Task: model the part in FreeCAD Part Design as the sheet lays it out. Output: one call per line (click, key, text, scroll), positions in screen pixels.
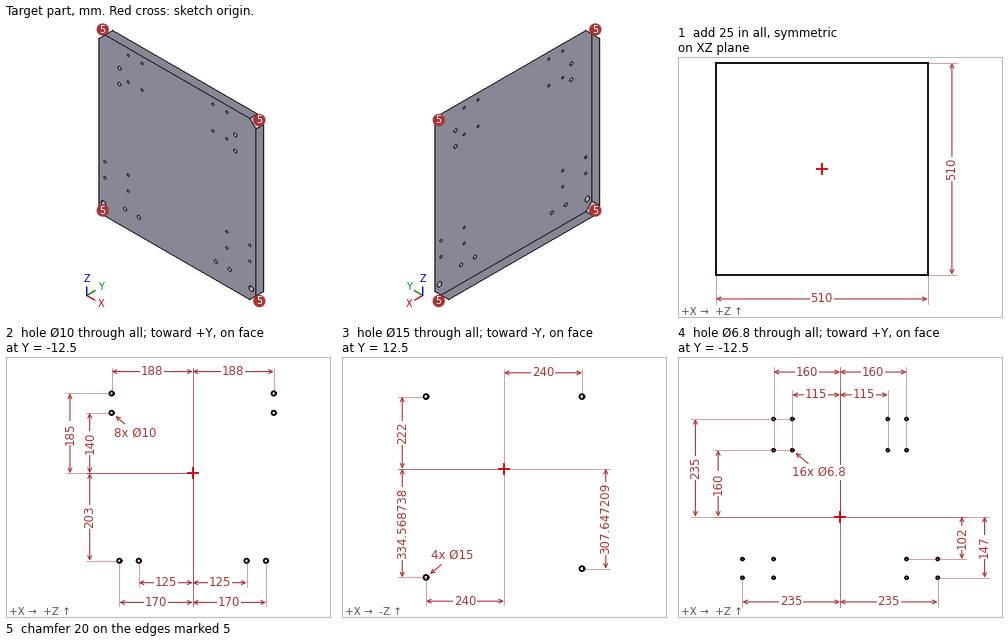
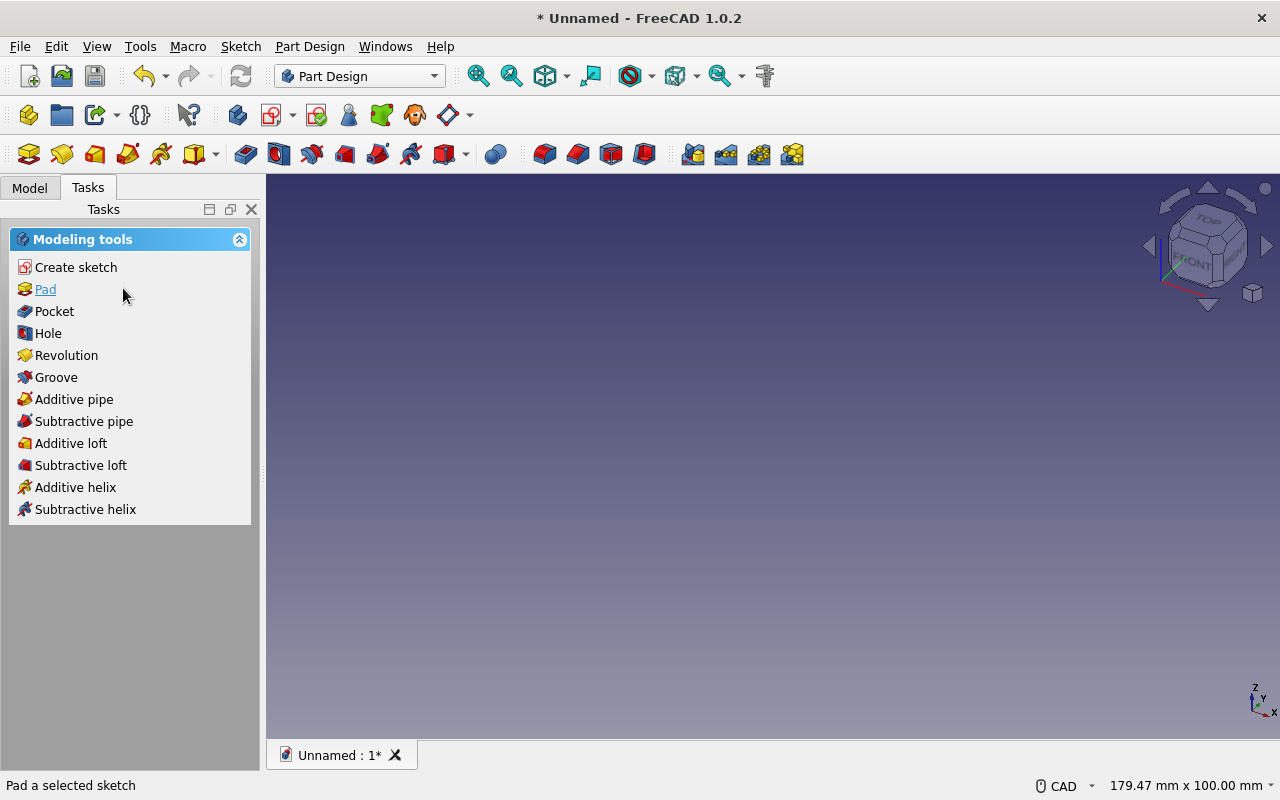
click(29, 154)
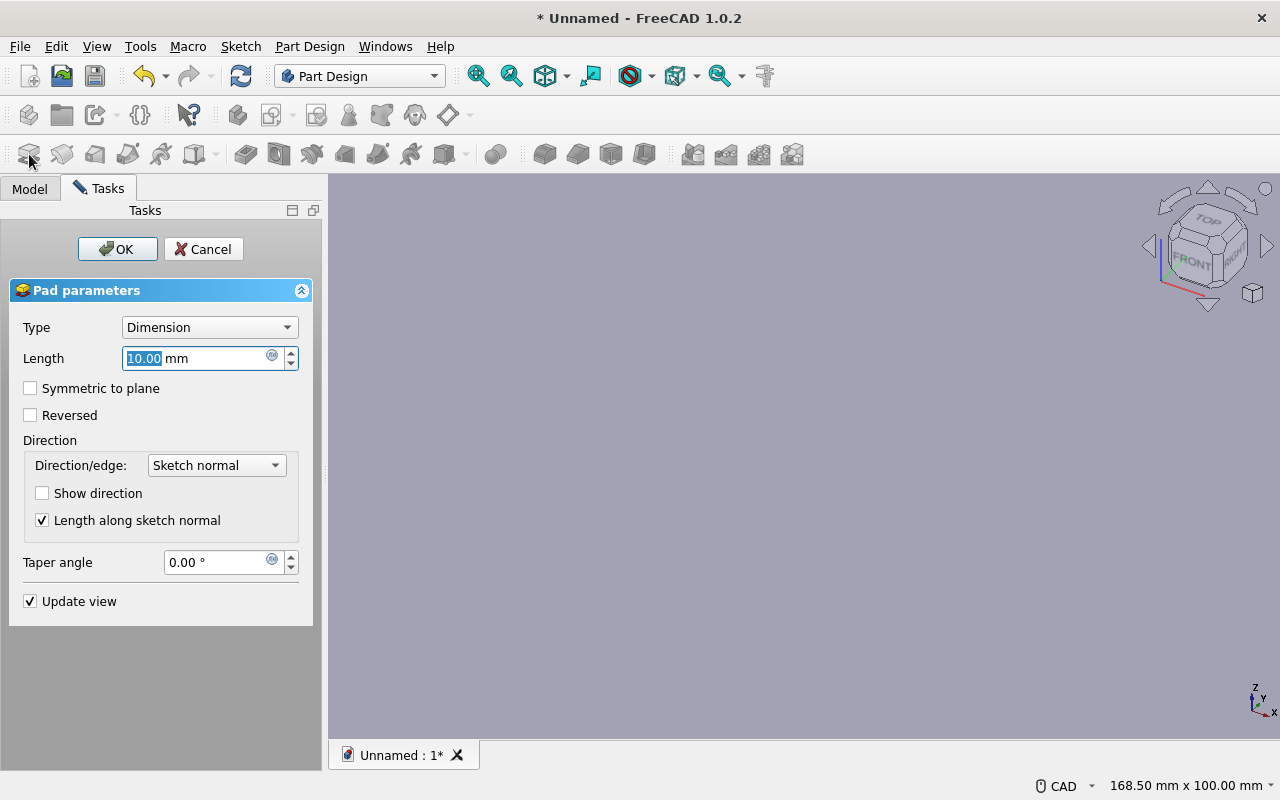
text(25)
key(Tab)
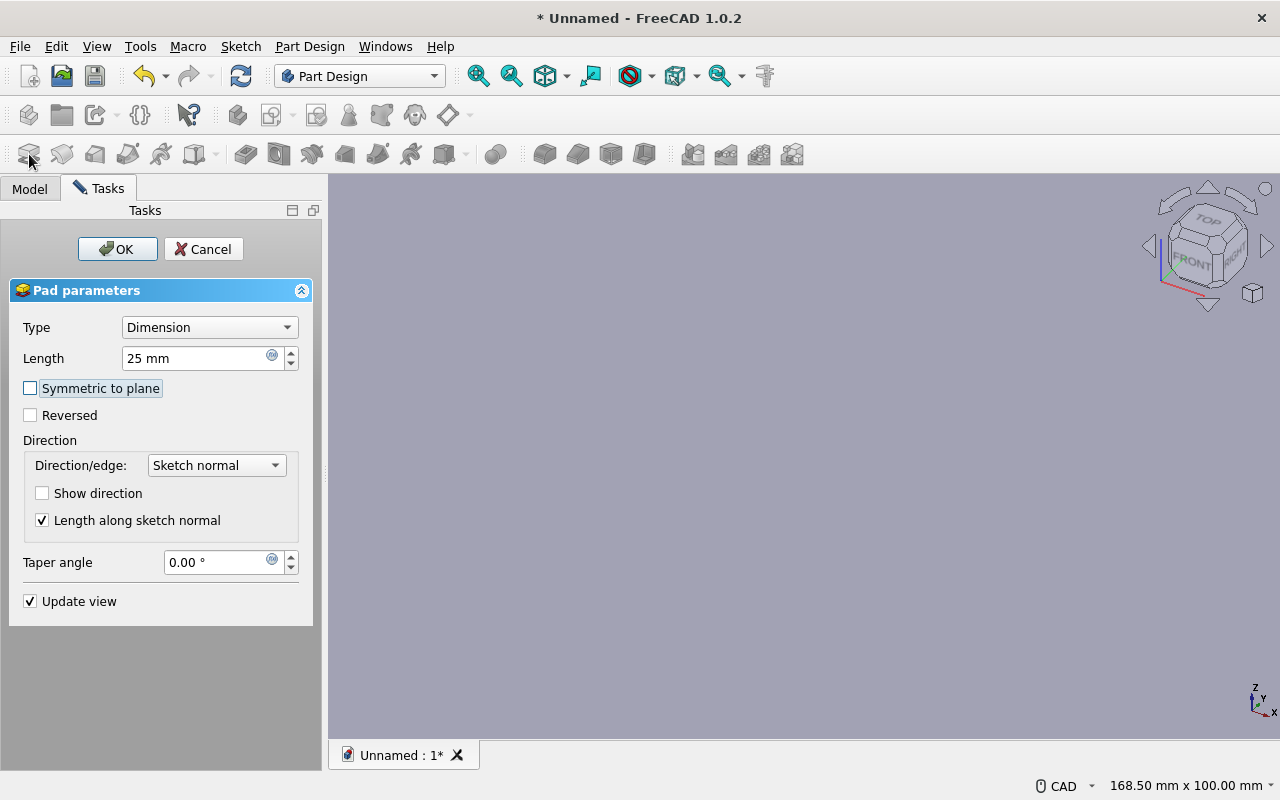
click(31, 388)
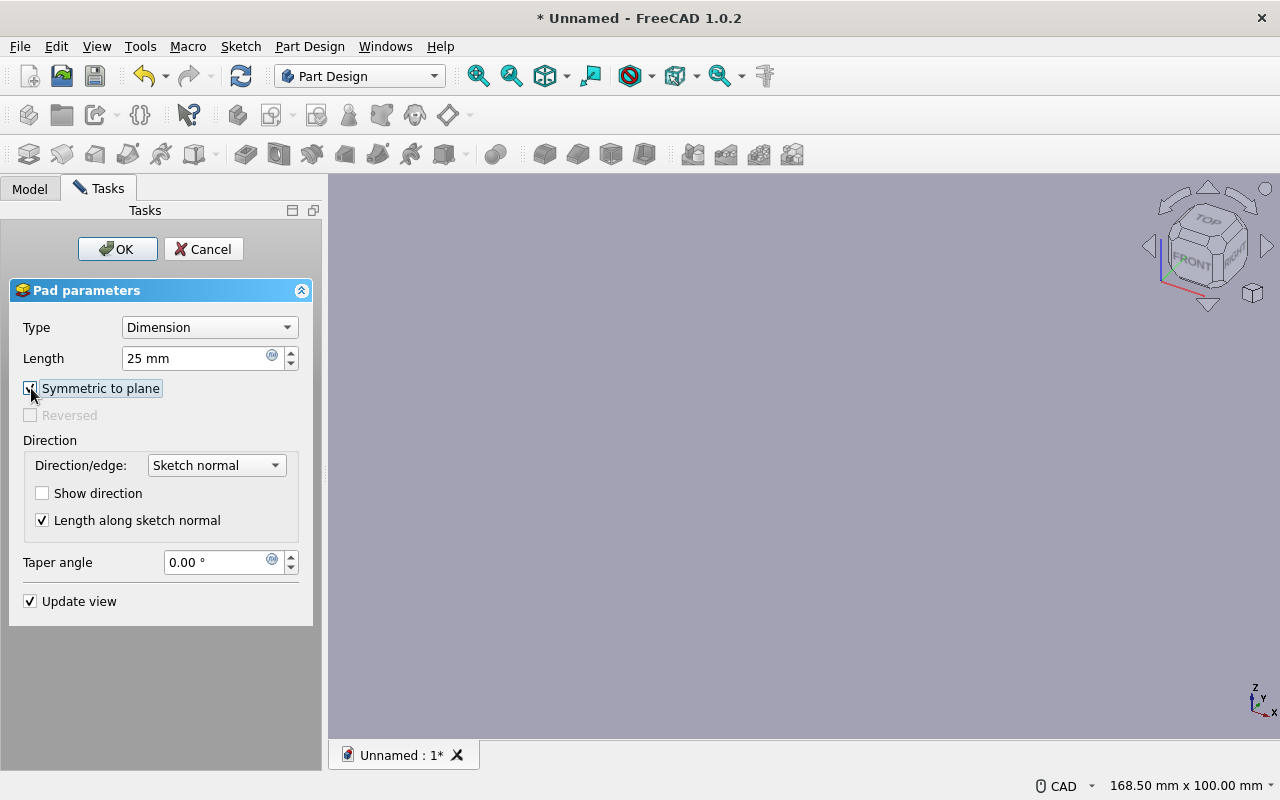
click(118, 249)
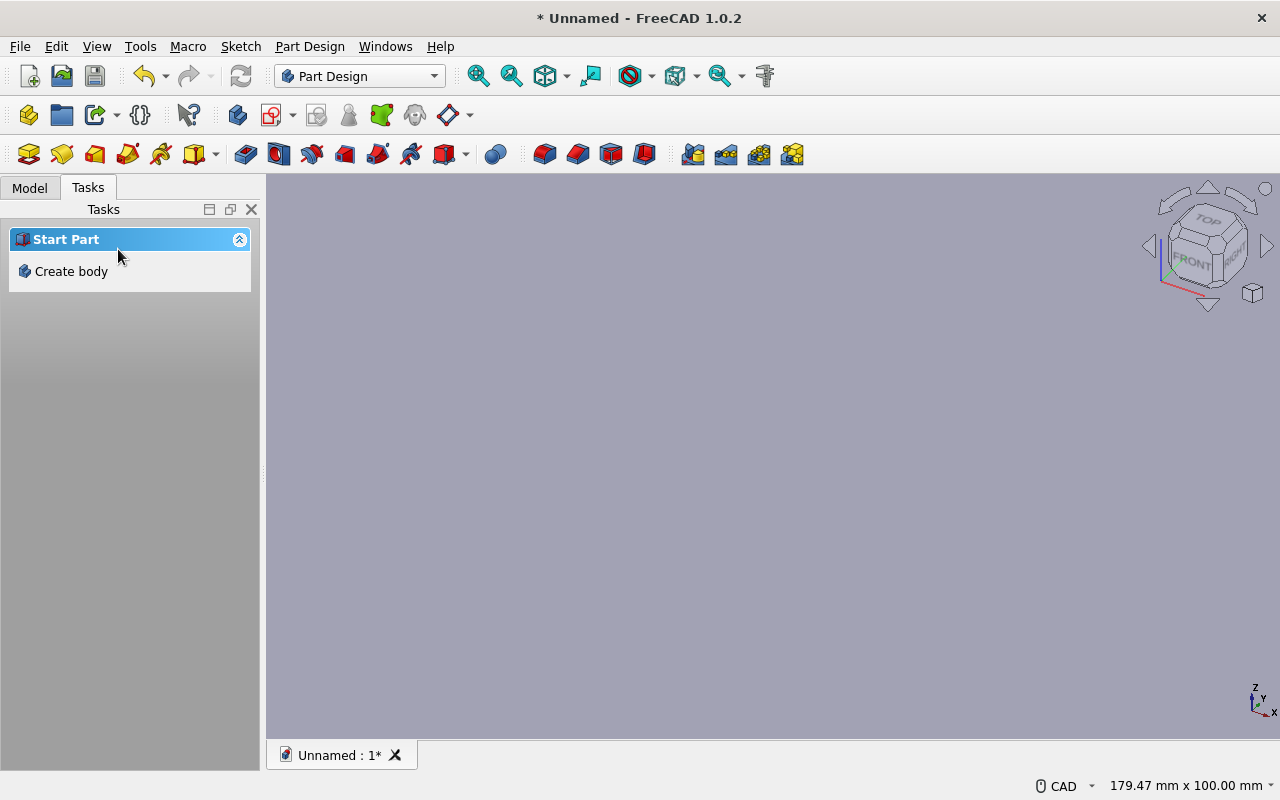
click(479, 76)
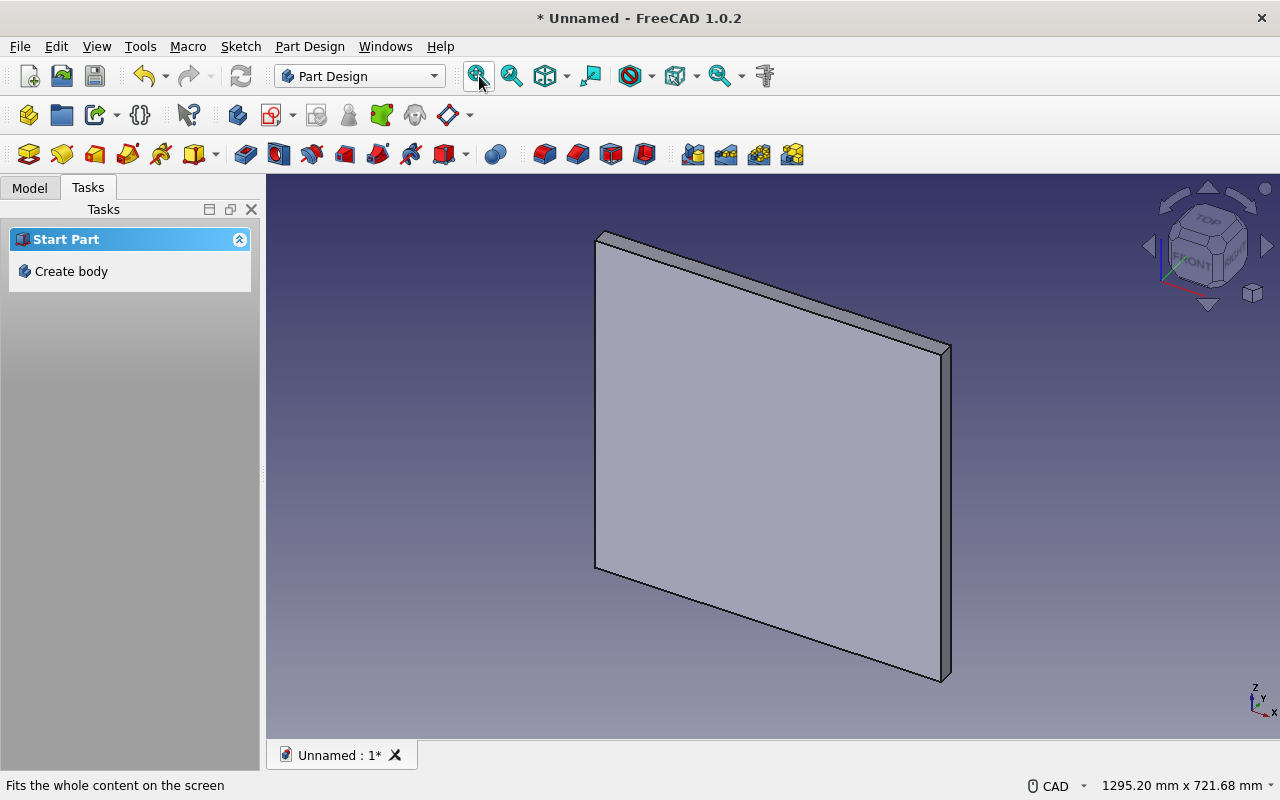
click(768, 460)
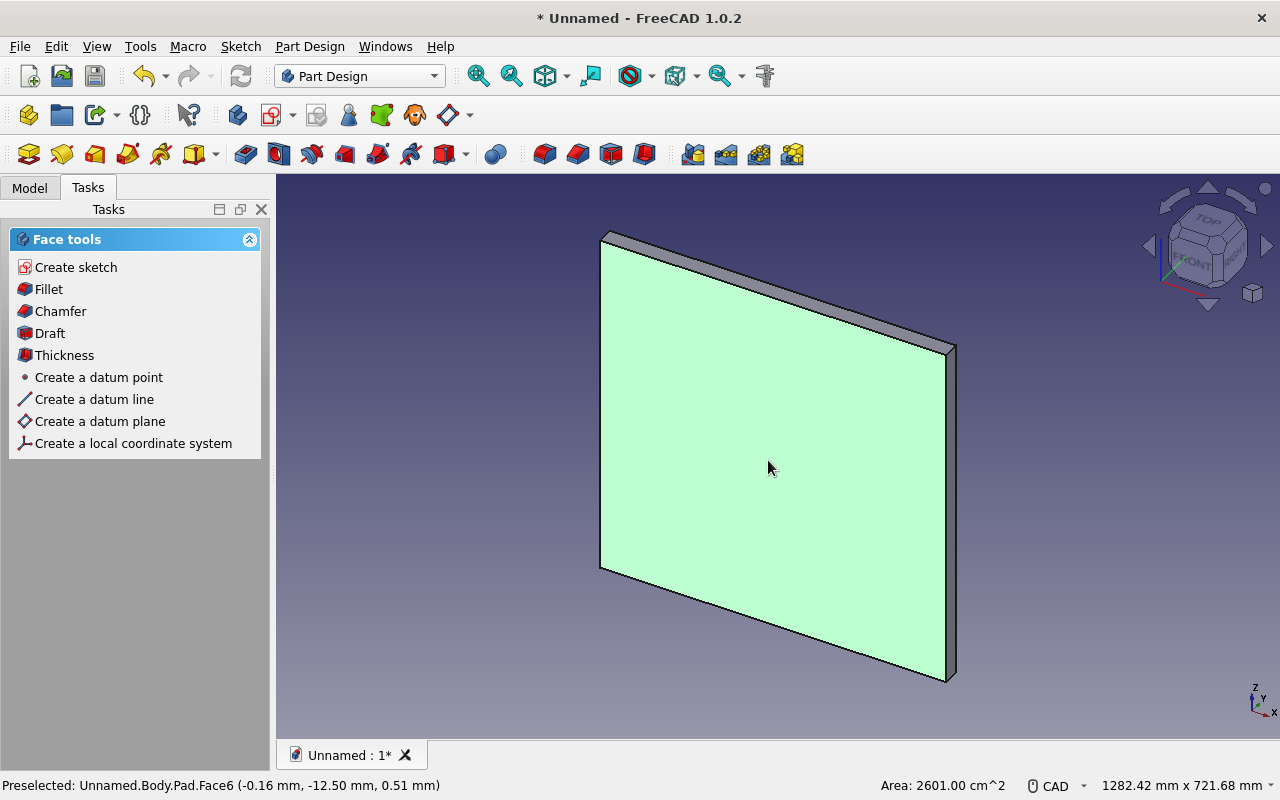
click(270, 116)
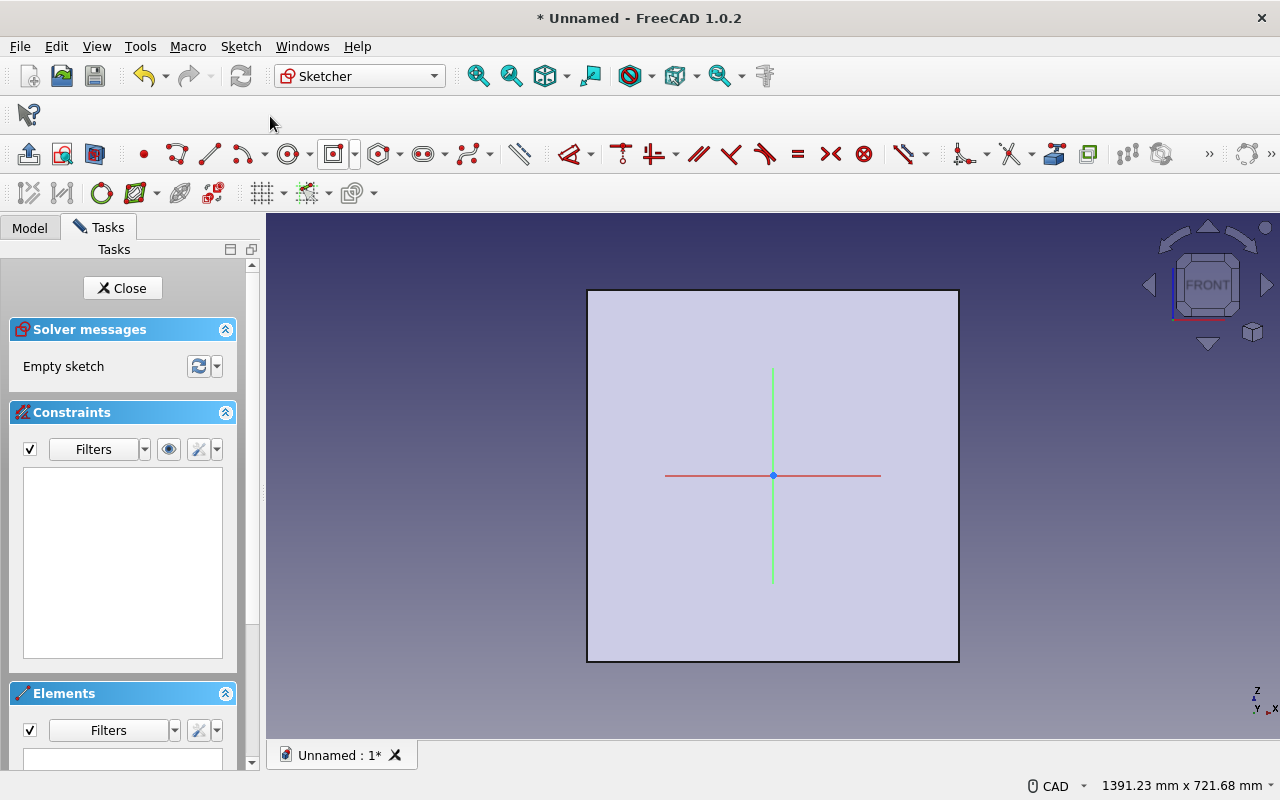
click(288, 154)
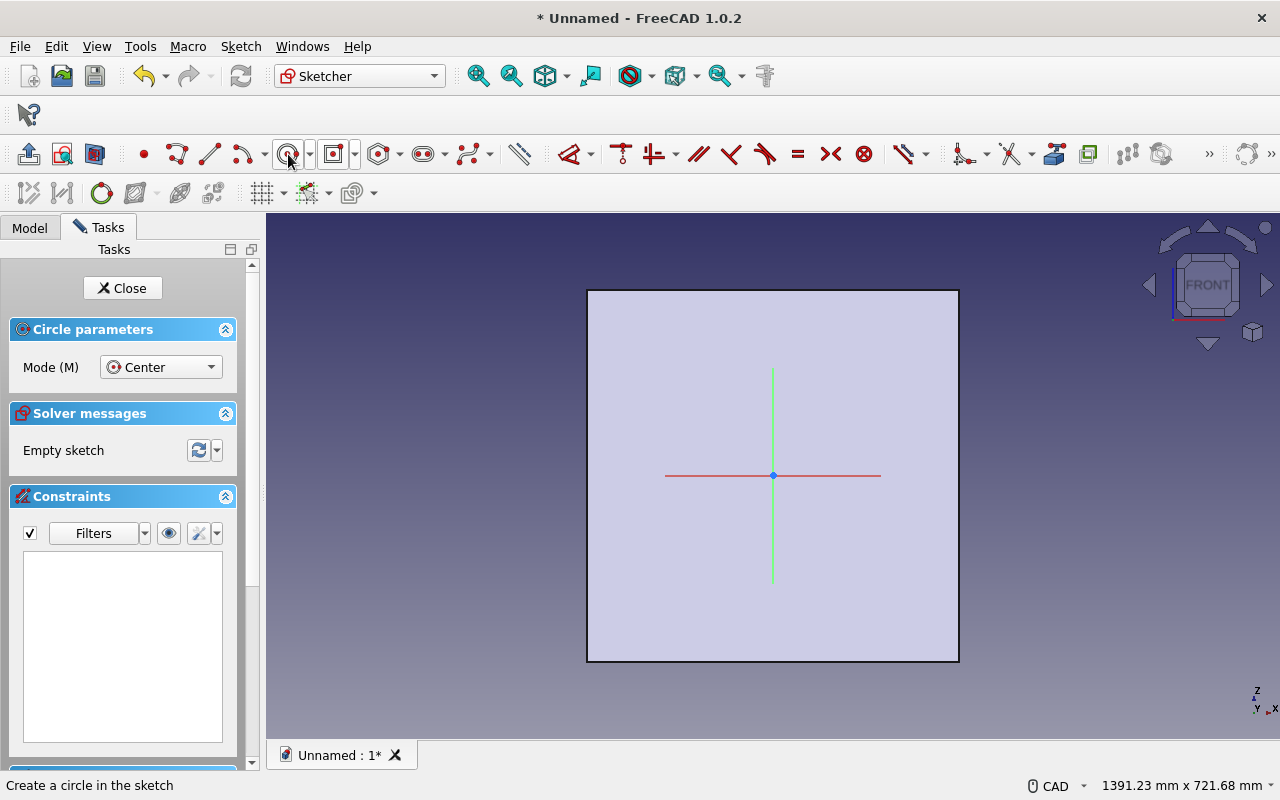
scroll(636, 341, up, 10)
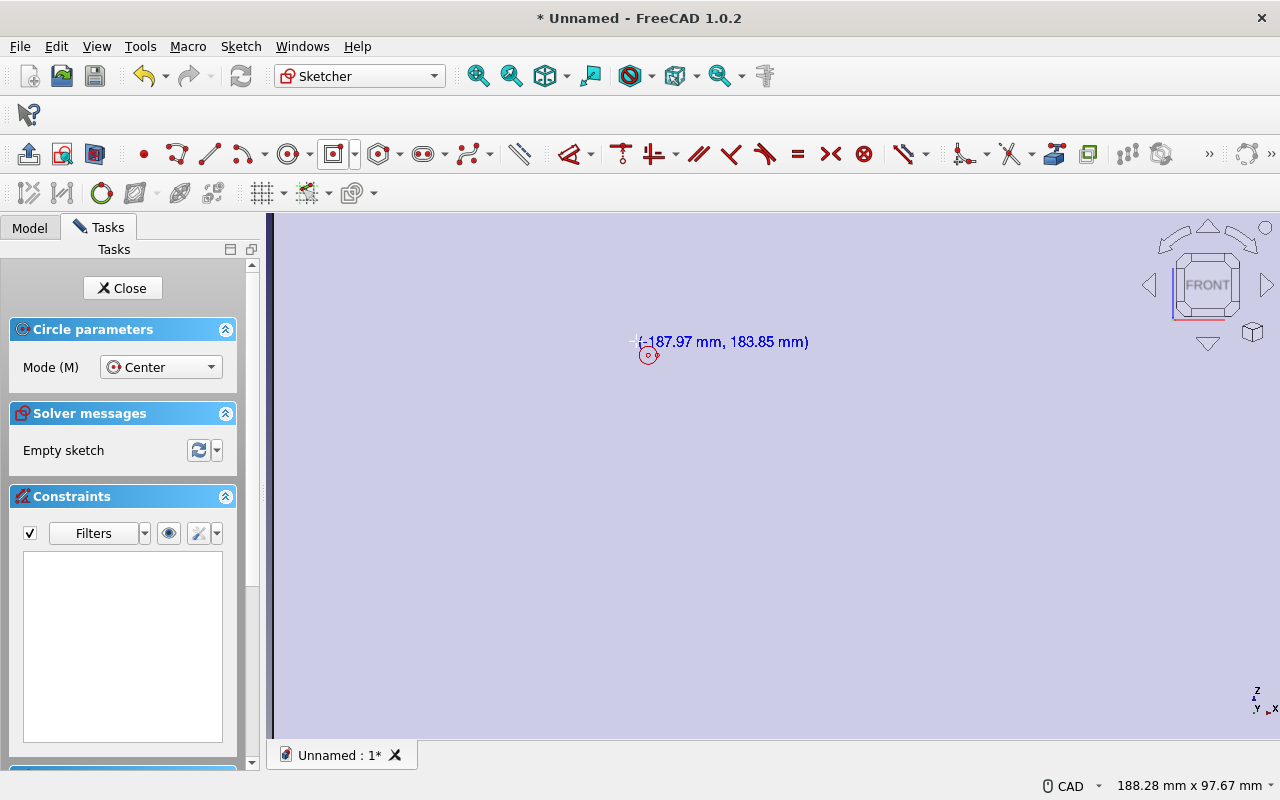
scroll(518, 296, down, 9)